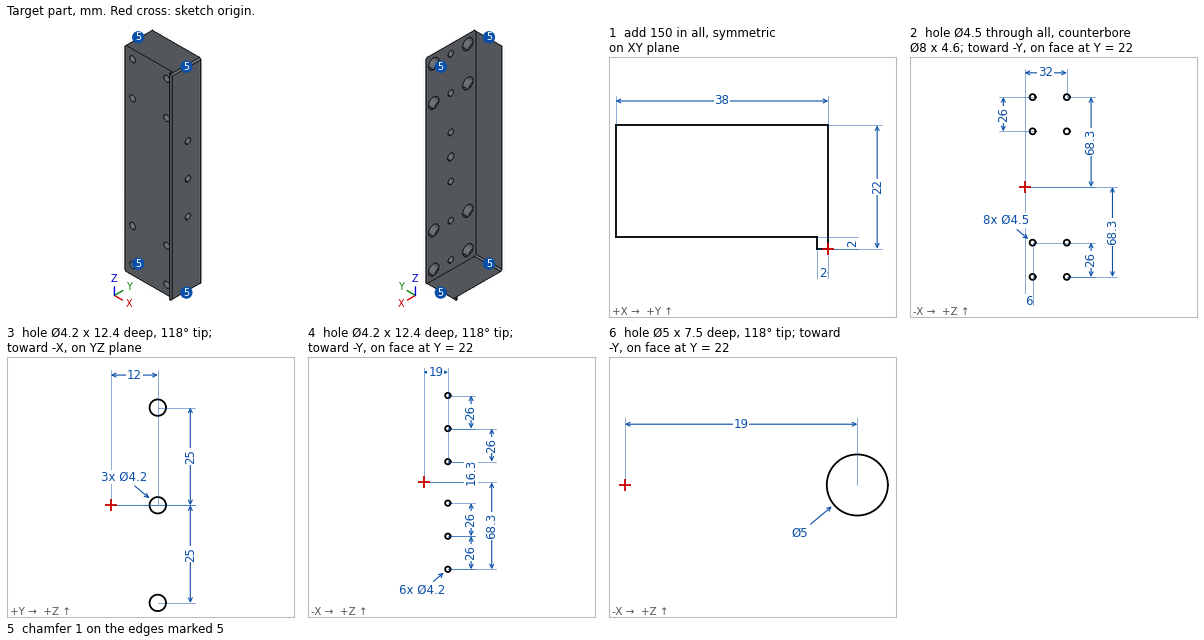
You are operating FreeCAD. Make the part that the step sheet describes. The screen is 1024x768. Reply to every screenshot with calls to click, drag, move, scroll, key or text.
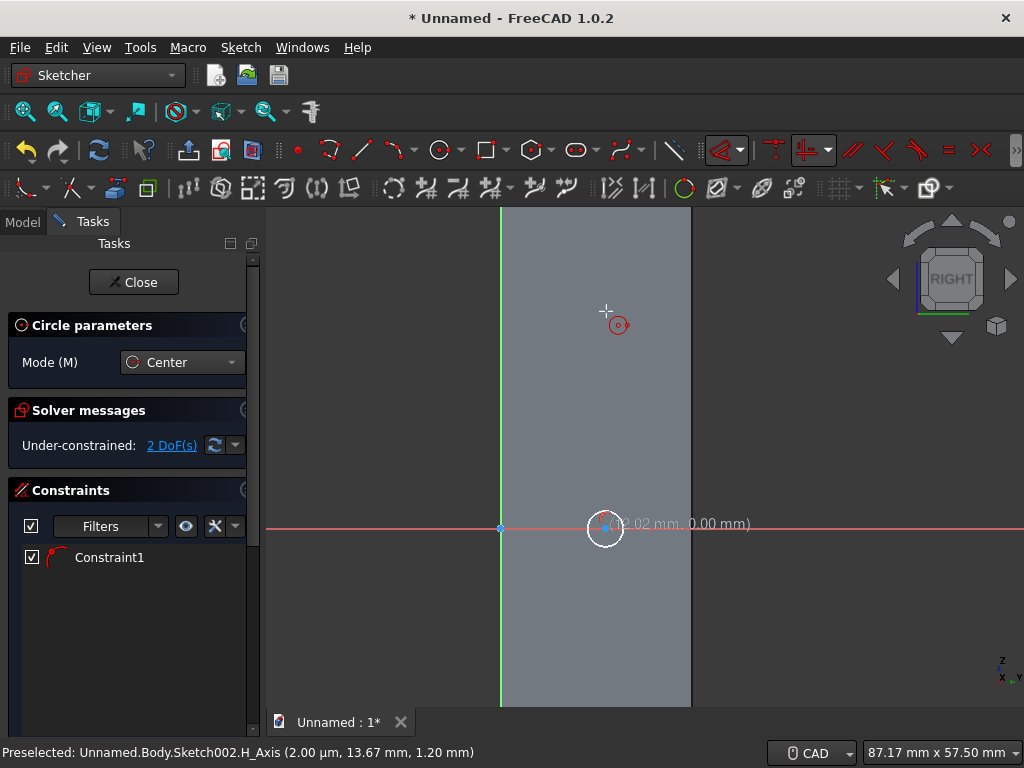
click(605, 312)
click(624, 292)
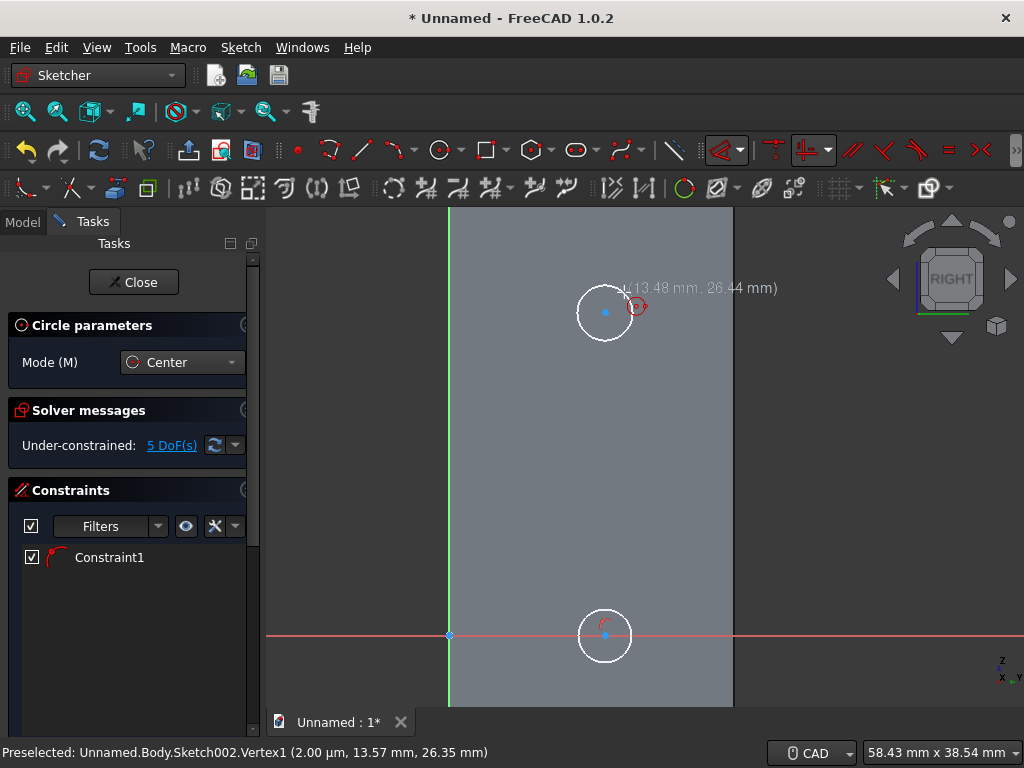
scroll(606, 311, down, 4)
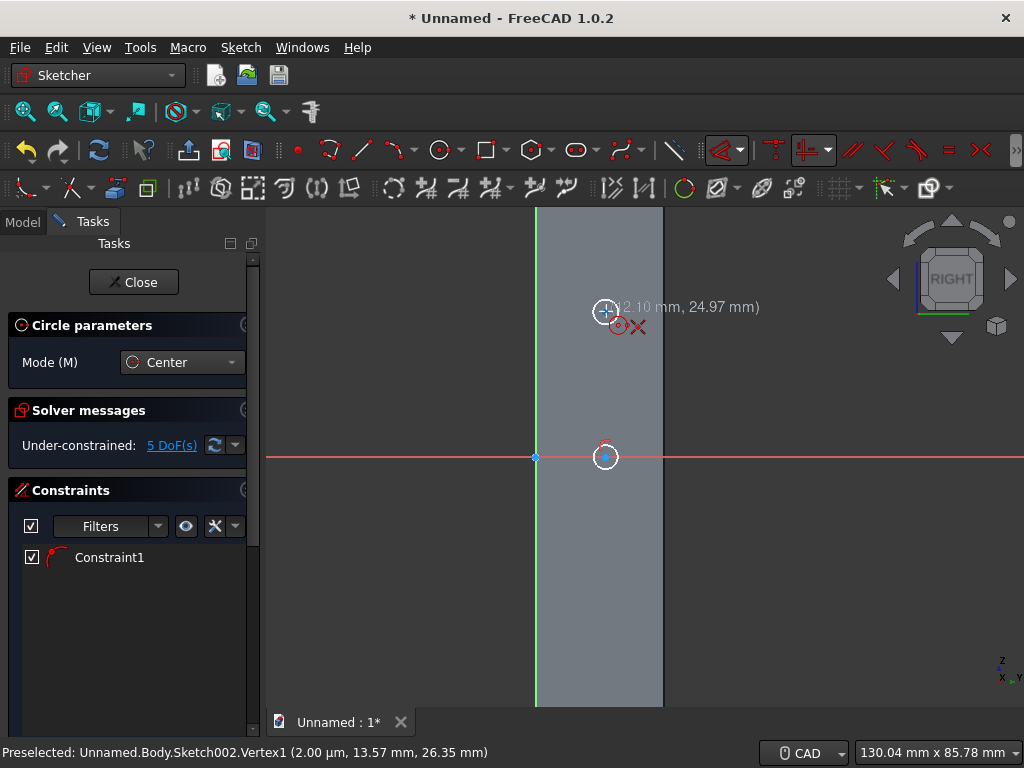
scroll(606, 603, up, 4)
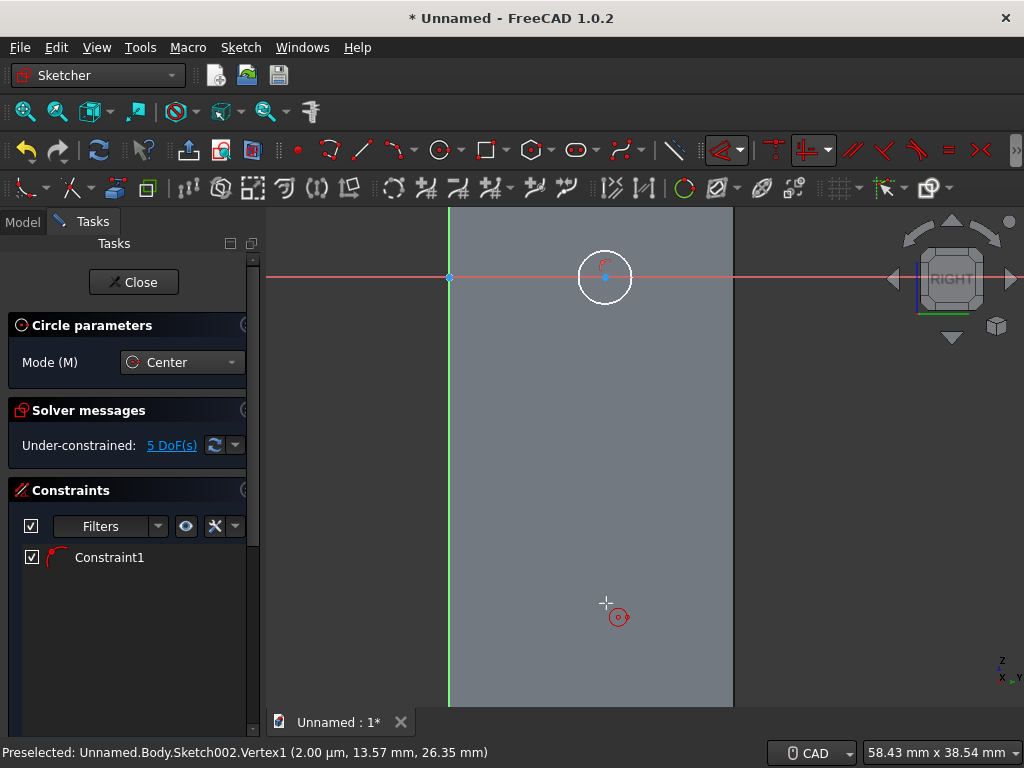
click(605, 602)
click(624, 582)
key(Escape)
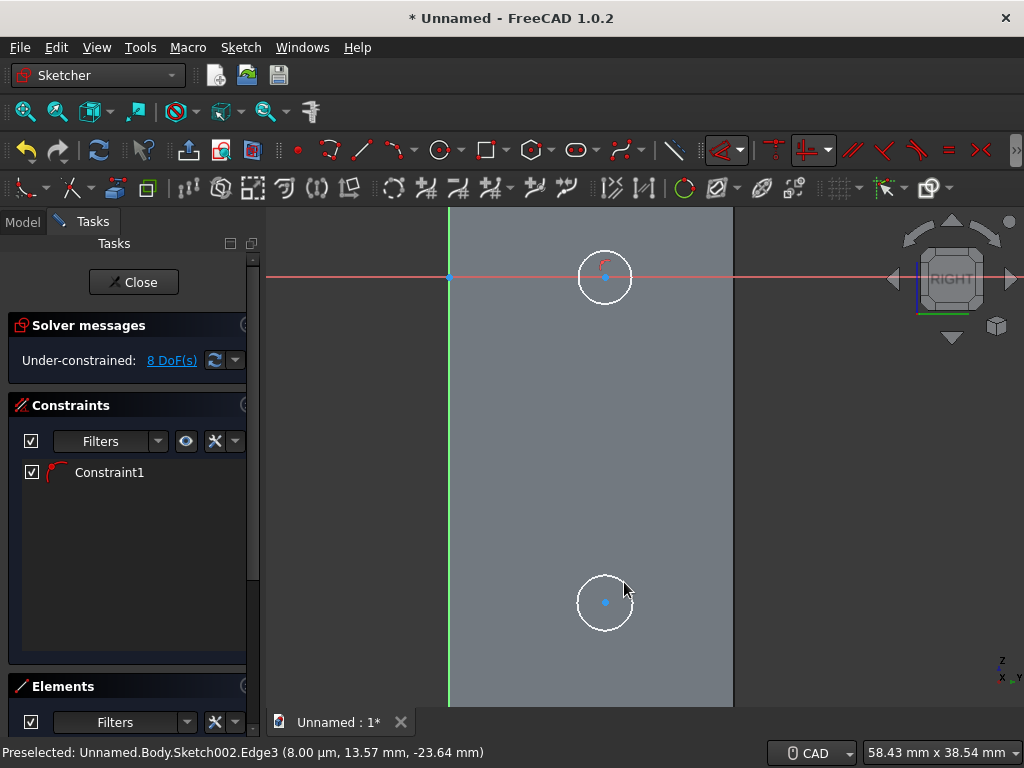
click(624, 259)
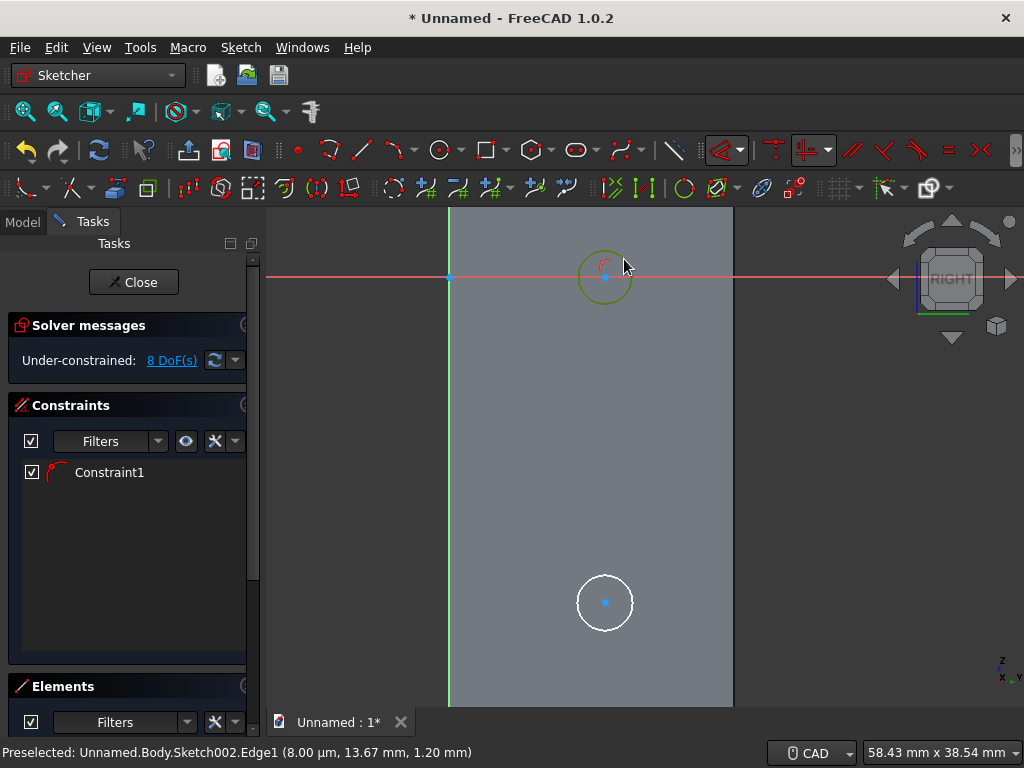
scroll(606, 604, down, 4)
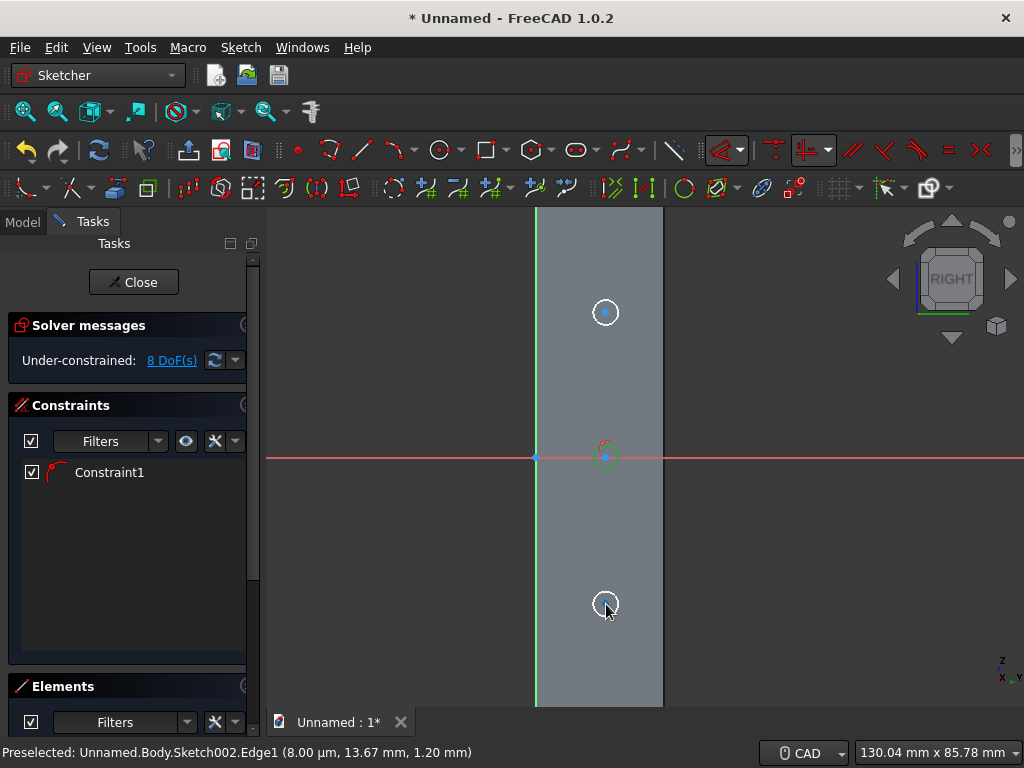
click(615, 304)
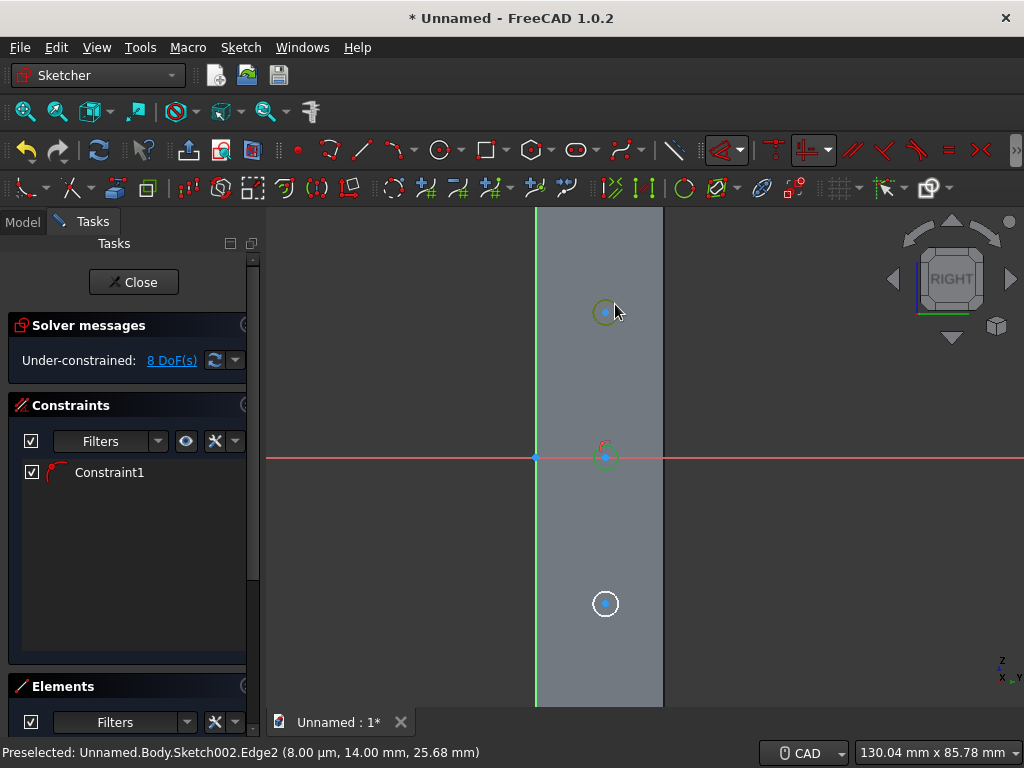
click(615, 595)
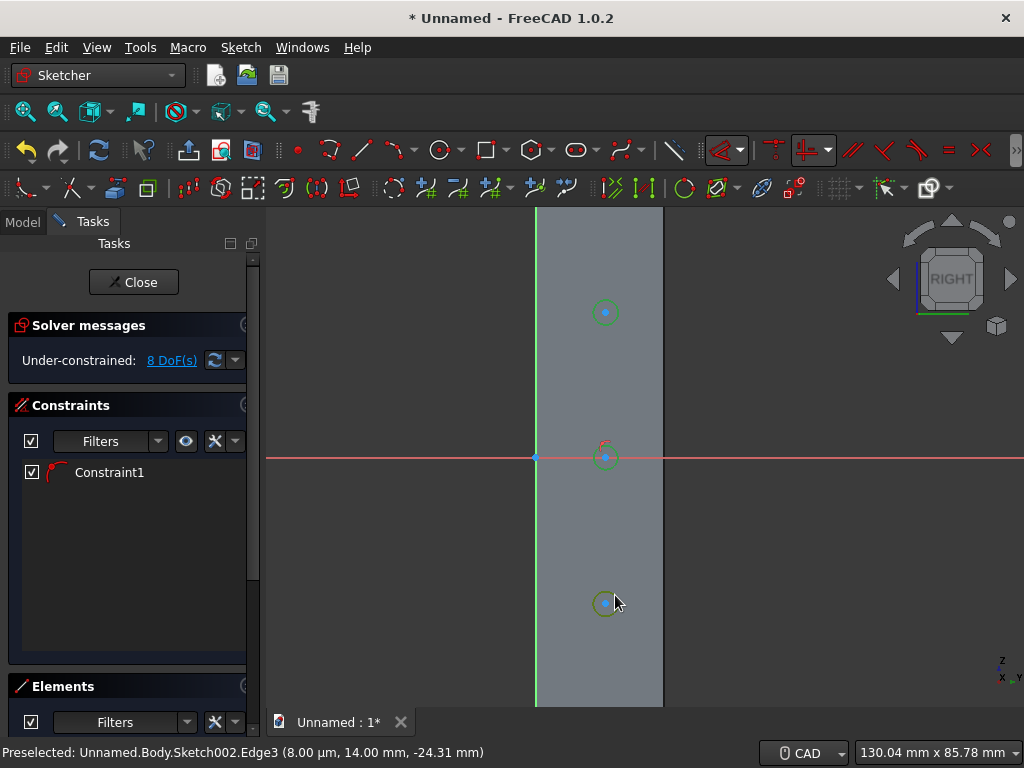
key(e)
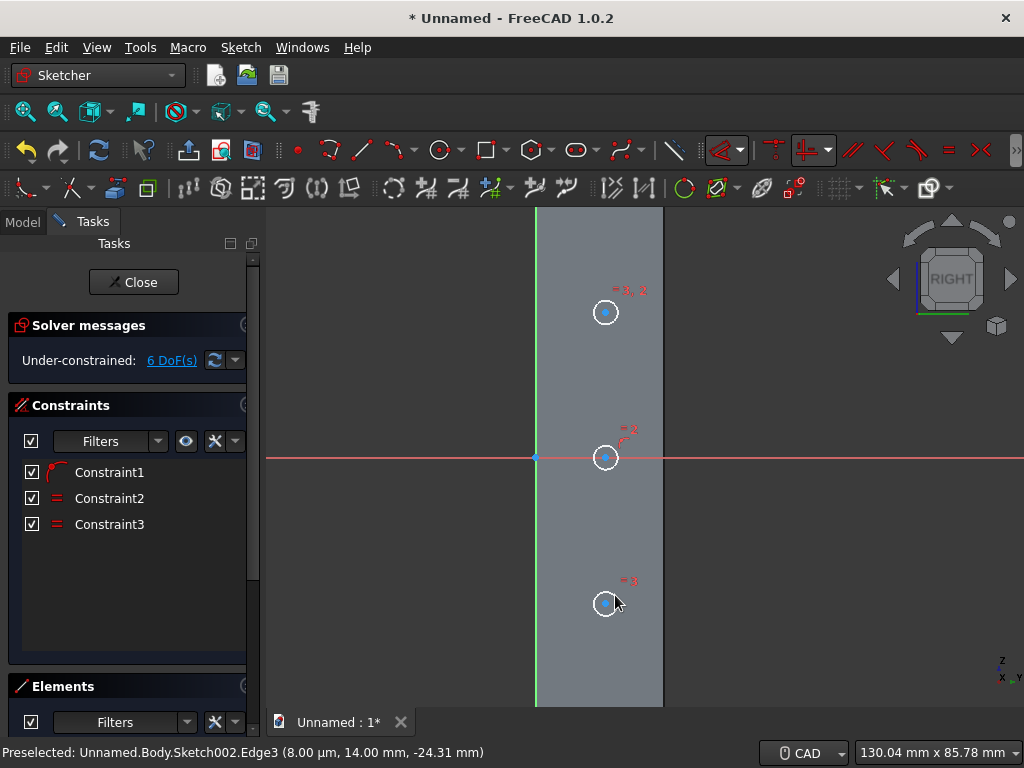
click(606, 458)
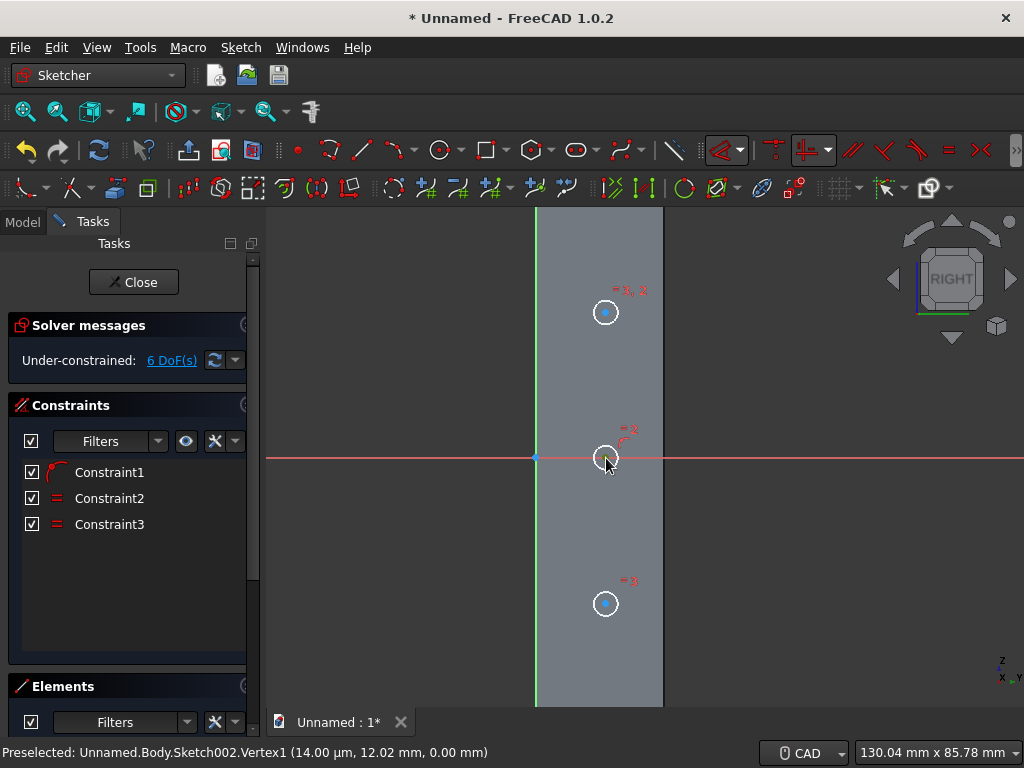
click(606, 313)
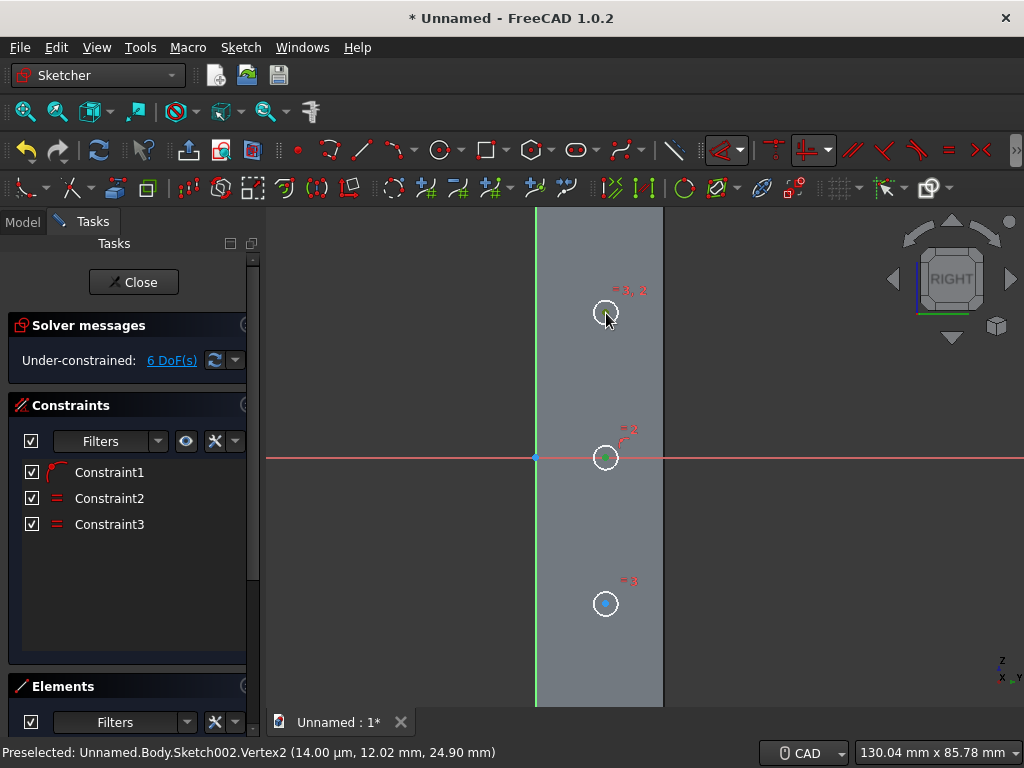
key(v)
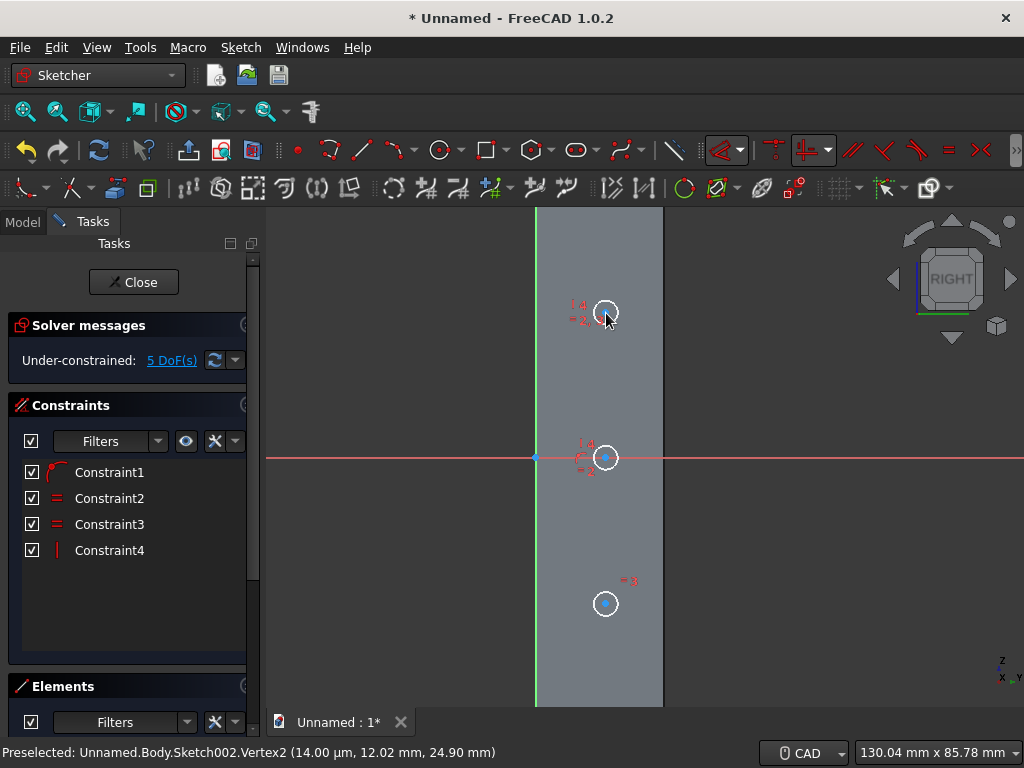
click(606, 458)